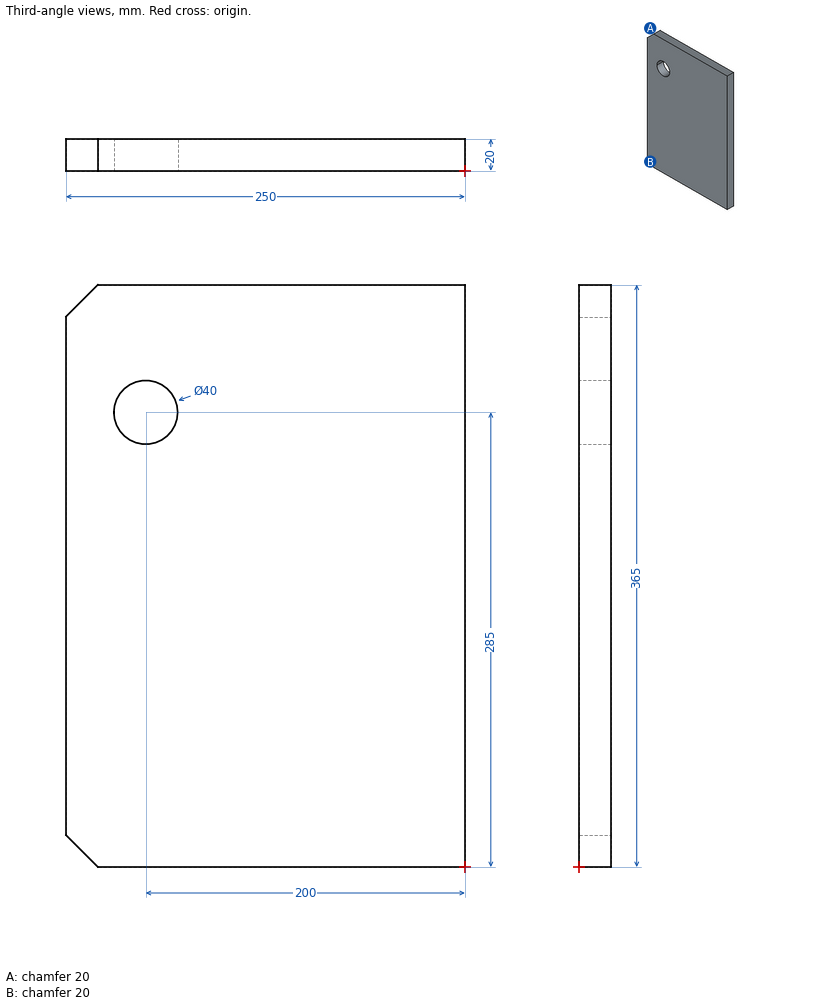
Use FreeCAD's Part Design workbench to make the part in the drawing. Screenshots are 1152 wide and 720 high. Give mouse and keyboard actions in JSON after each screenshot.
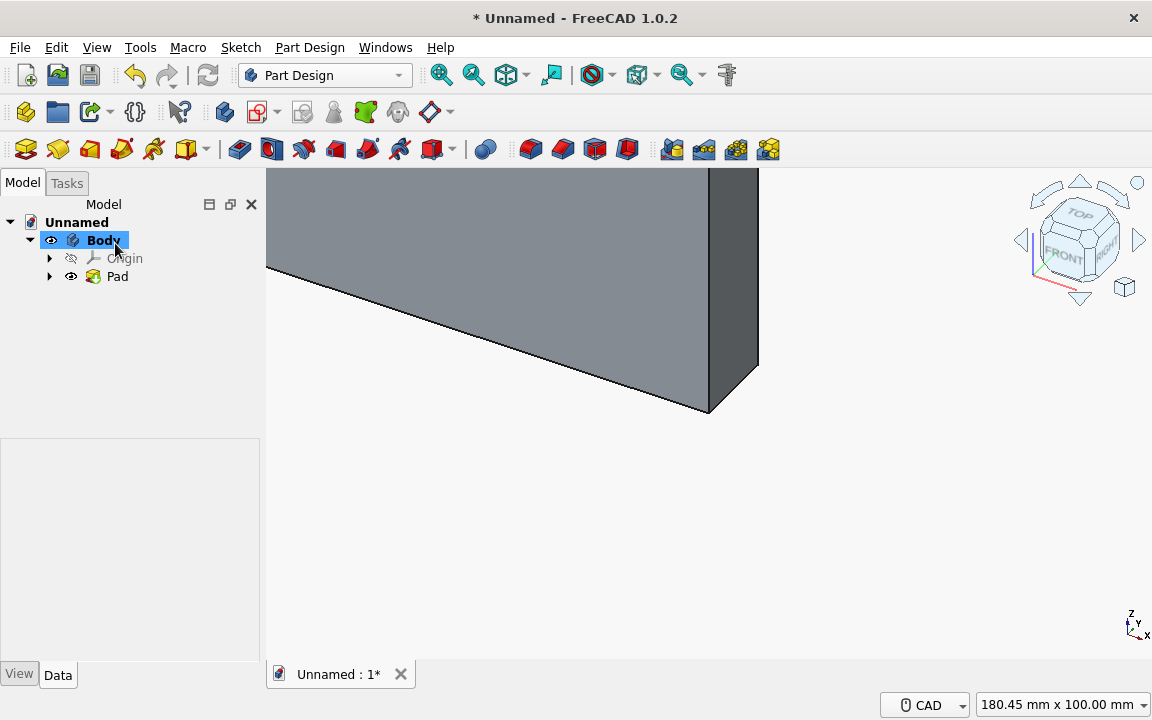
{"action": "key", "text": "v f"}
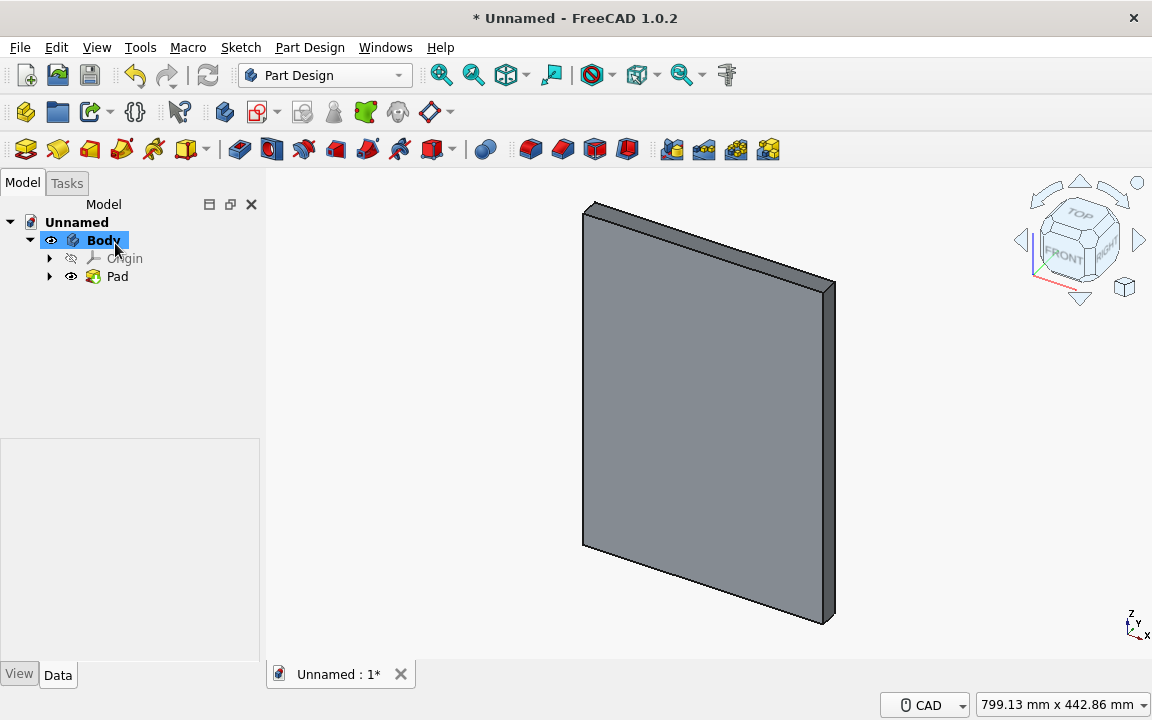
{"action": "key", "text": "0"}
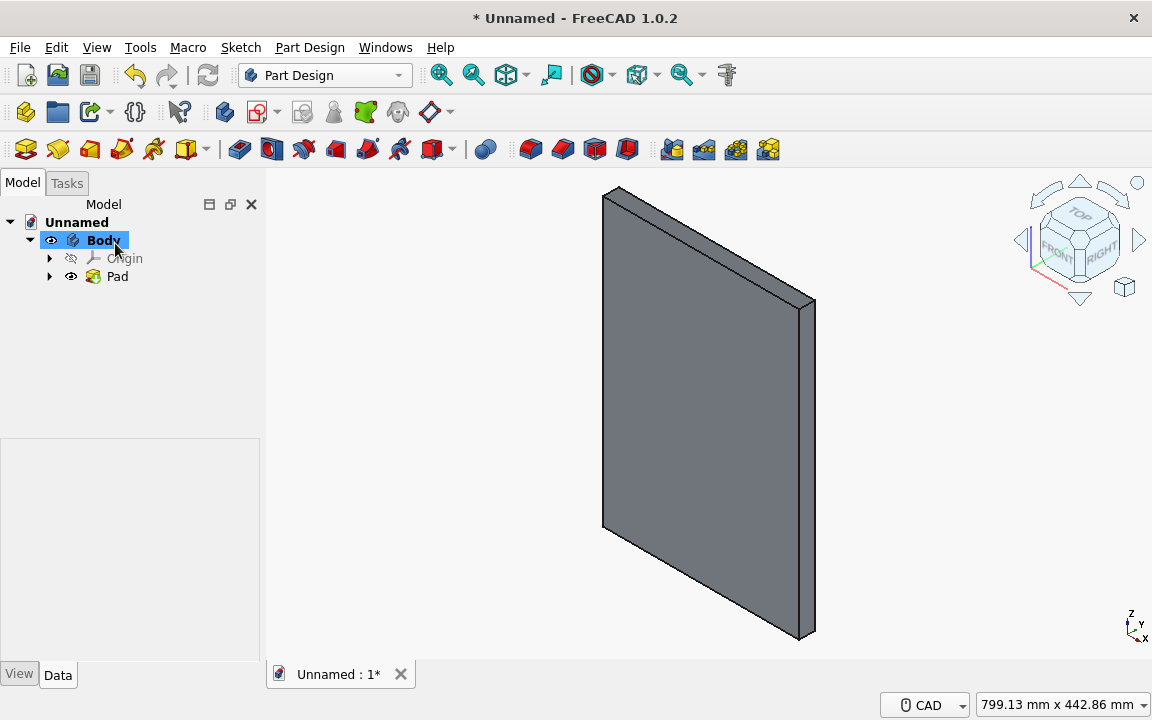
{"action": "key", "text": "2"}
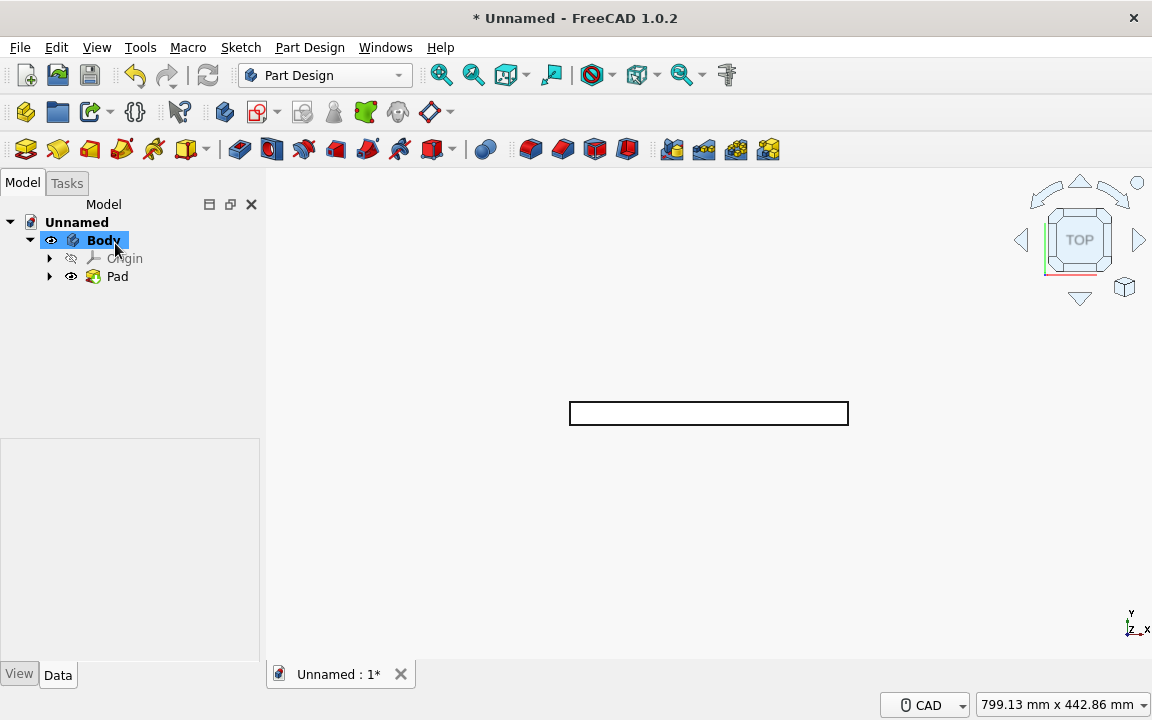
{"action": "key", "text": "v f"}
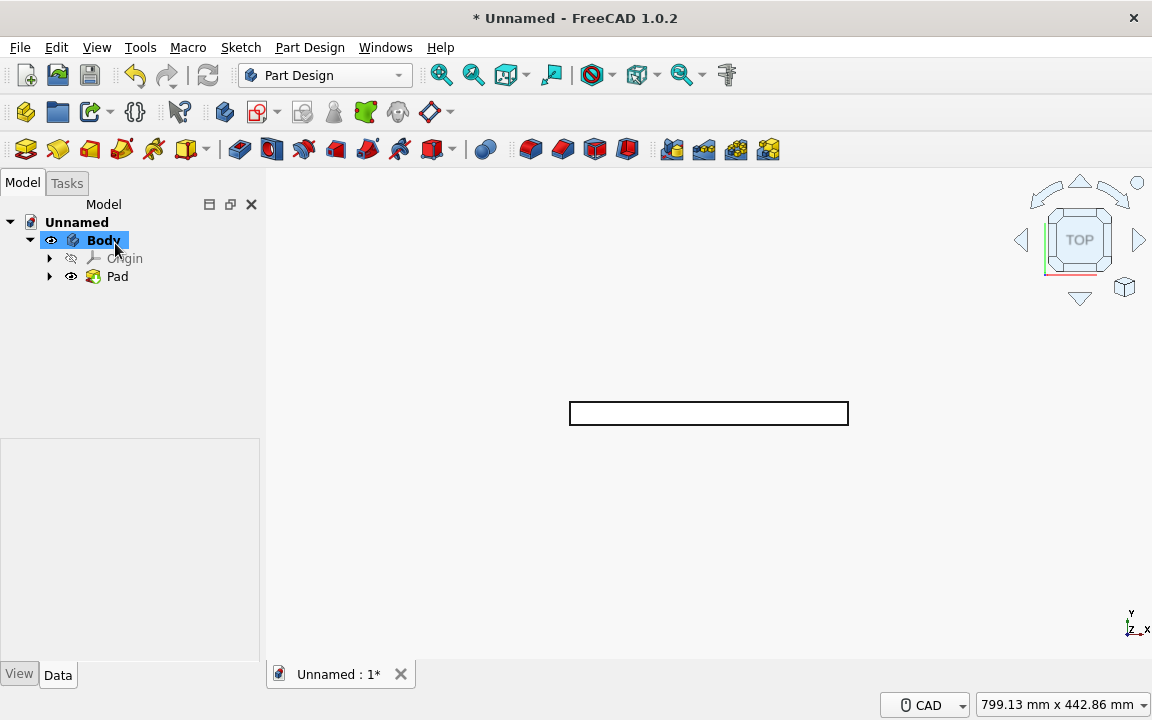
{"action": "left_click", "coordinate": [570, 412]}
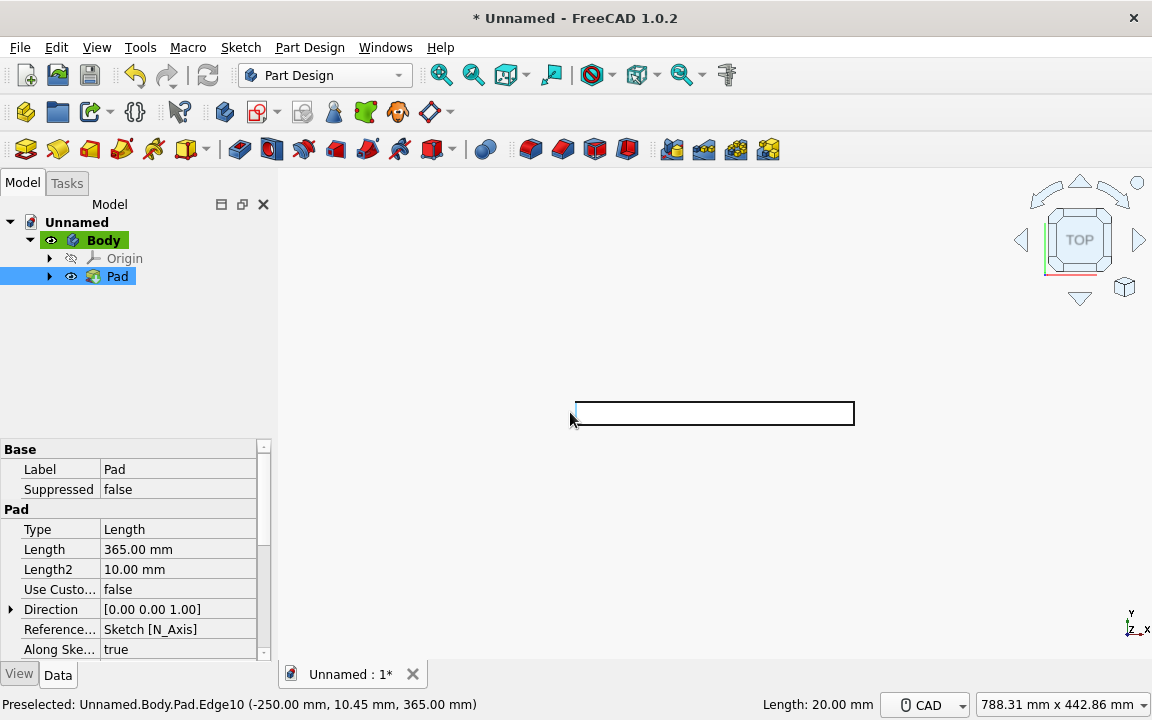
{"action": "left_click", "coordinate": [564, 150]}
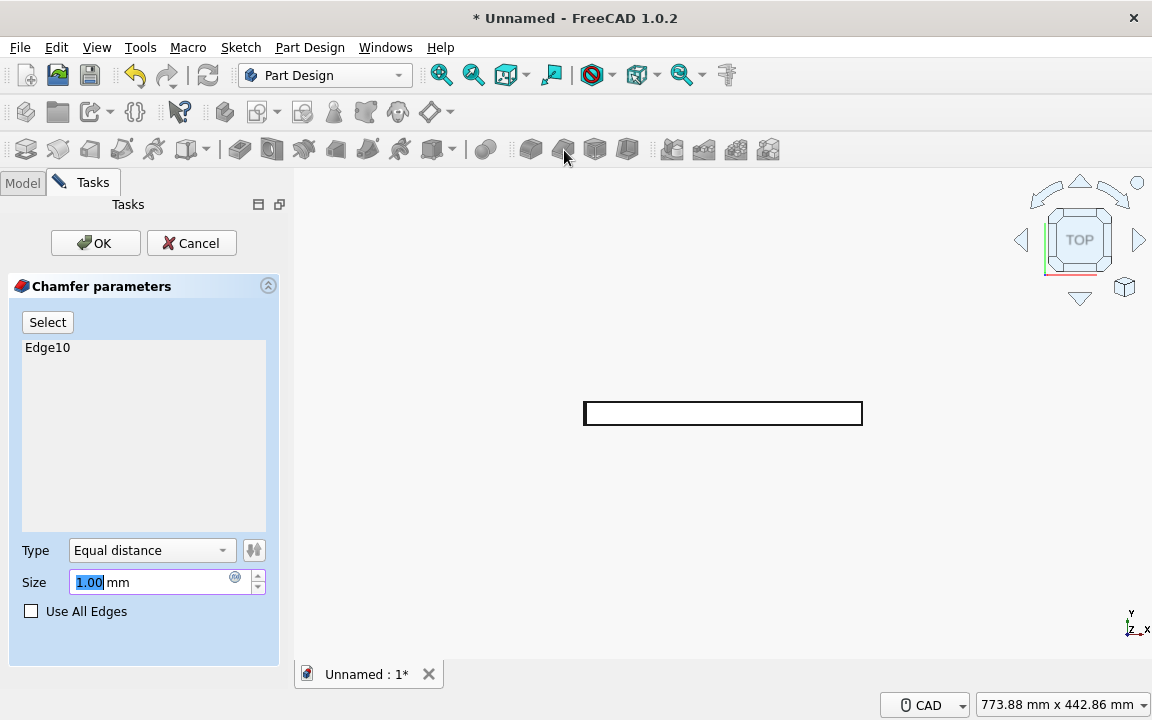
{"action": "type", "text": "20"}
{"action": "key", "text": "Tab"}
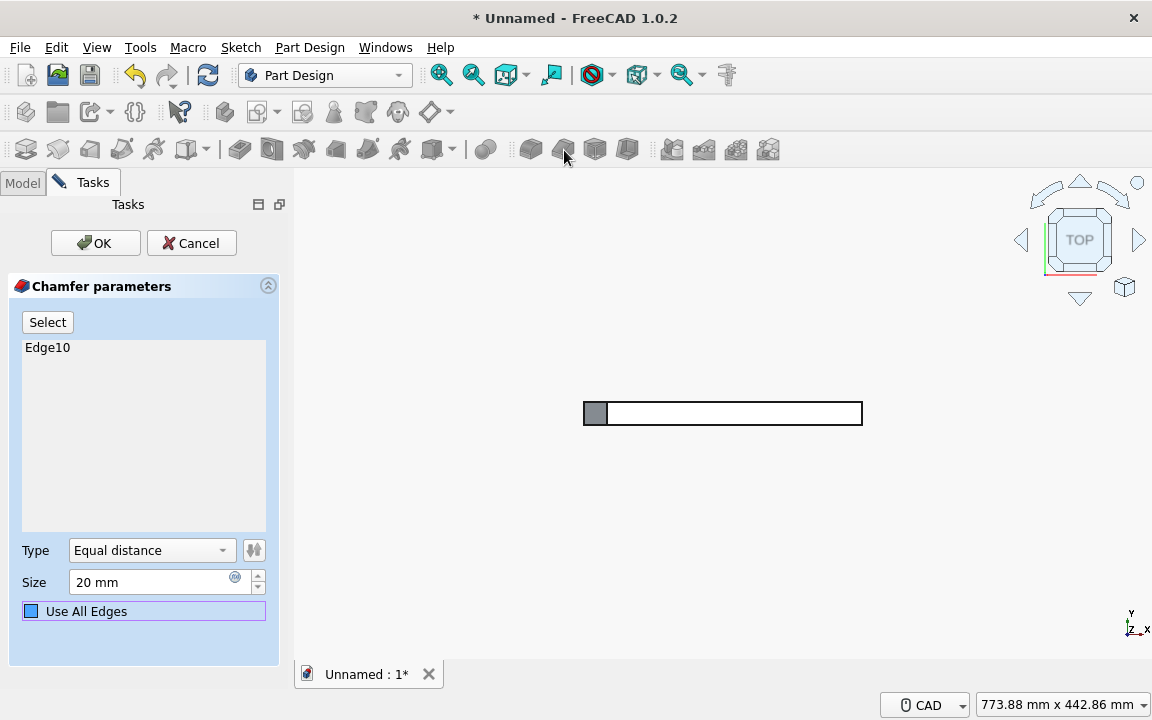
{"action": "left_click", "coordinate": [96, 243]}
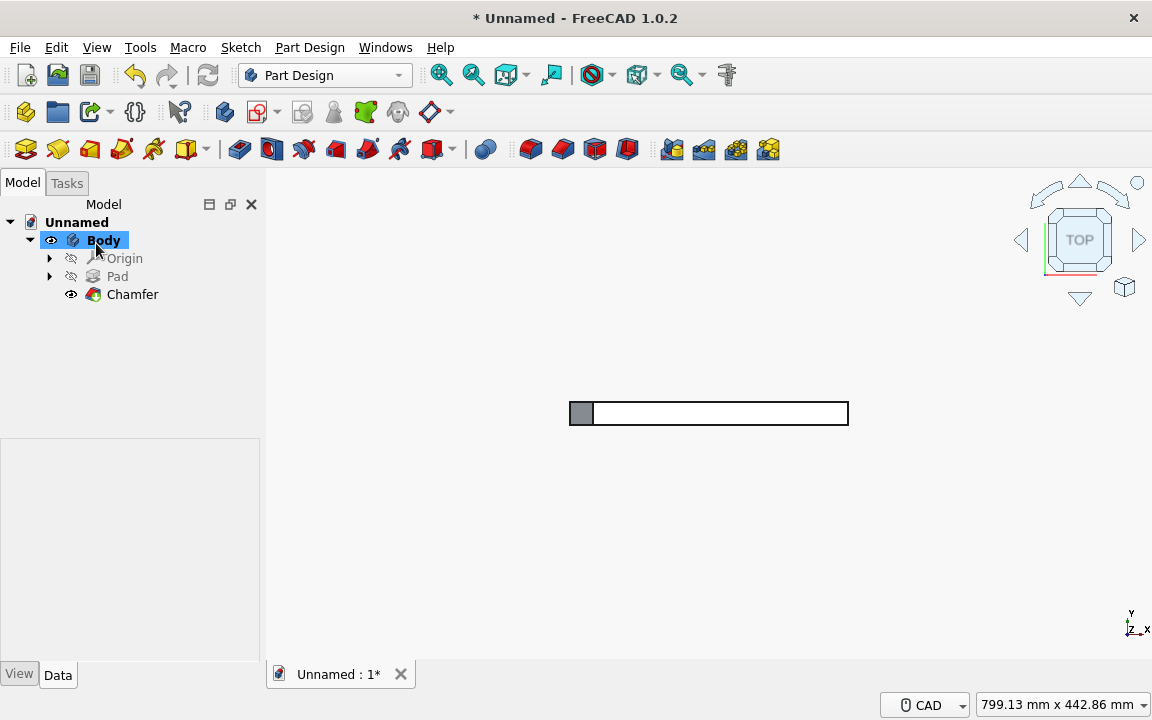
{"action": "key", "text": "v f"}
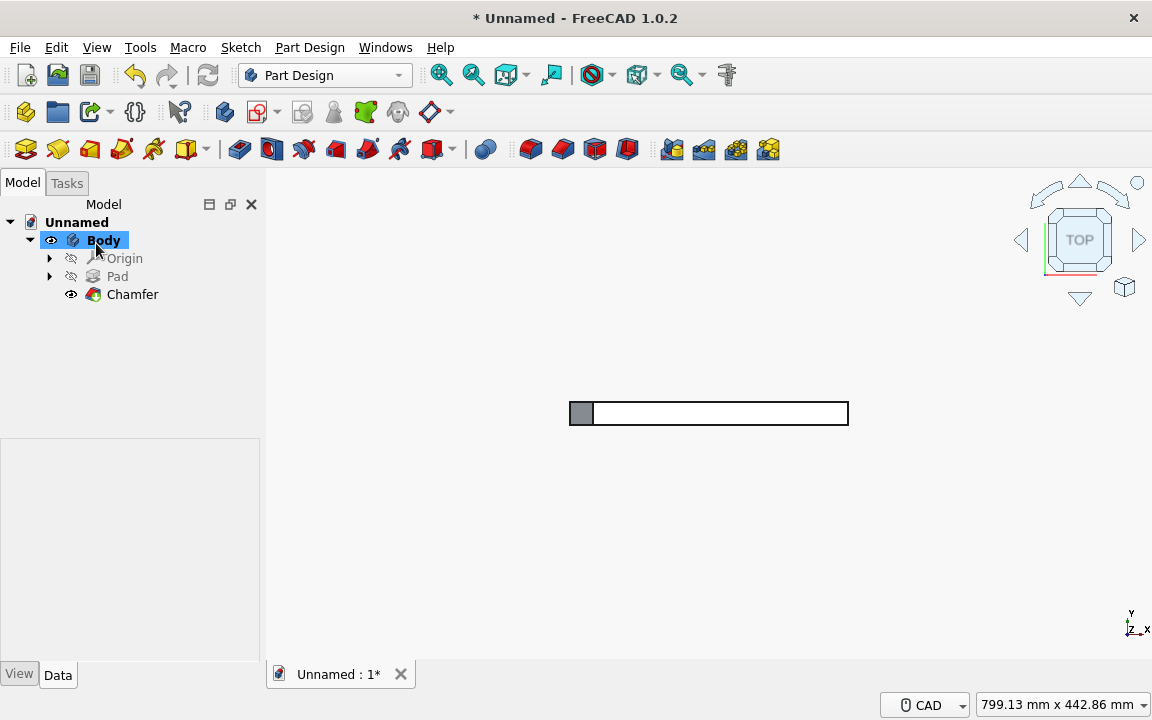
{"action": "key", "text": "4"}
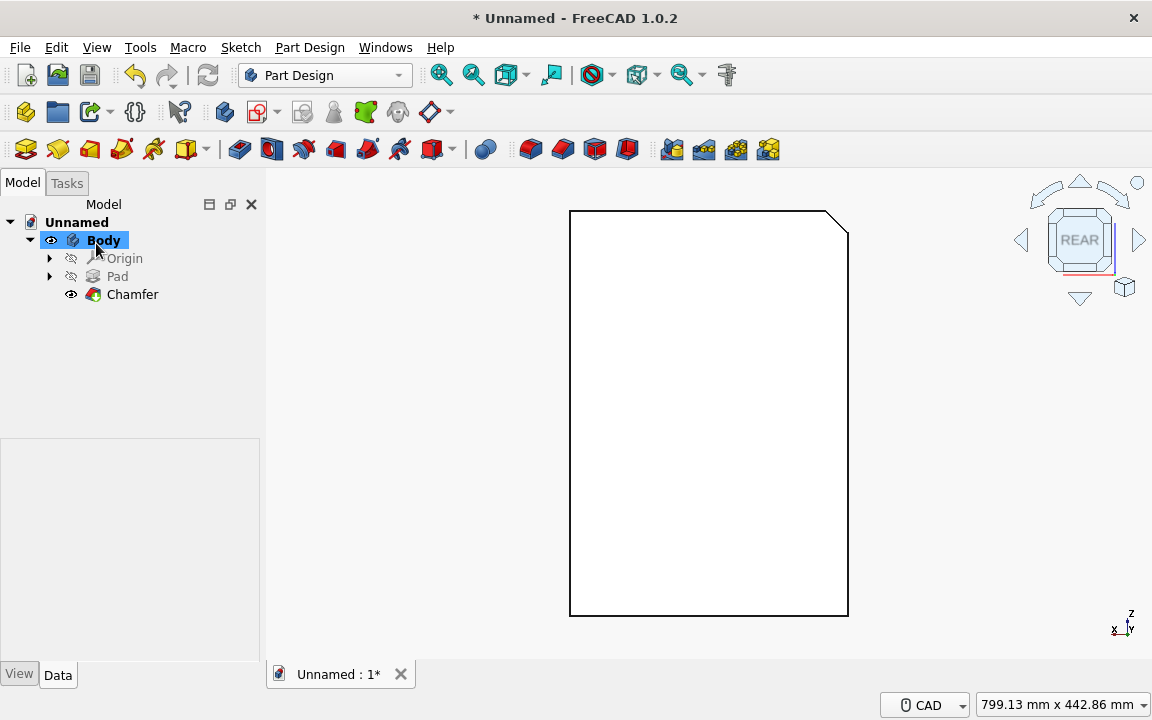
{"action": "left_click", "coordinate": [709, 355]}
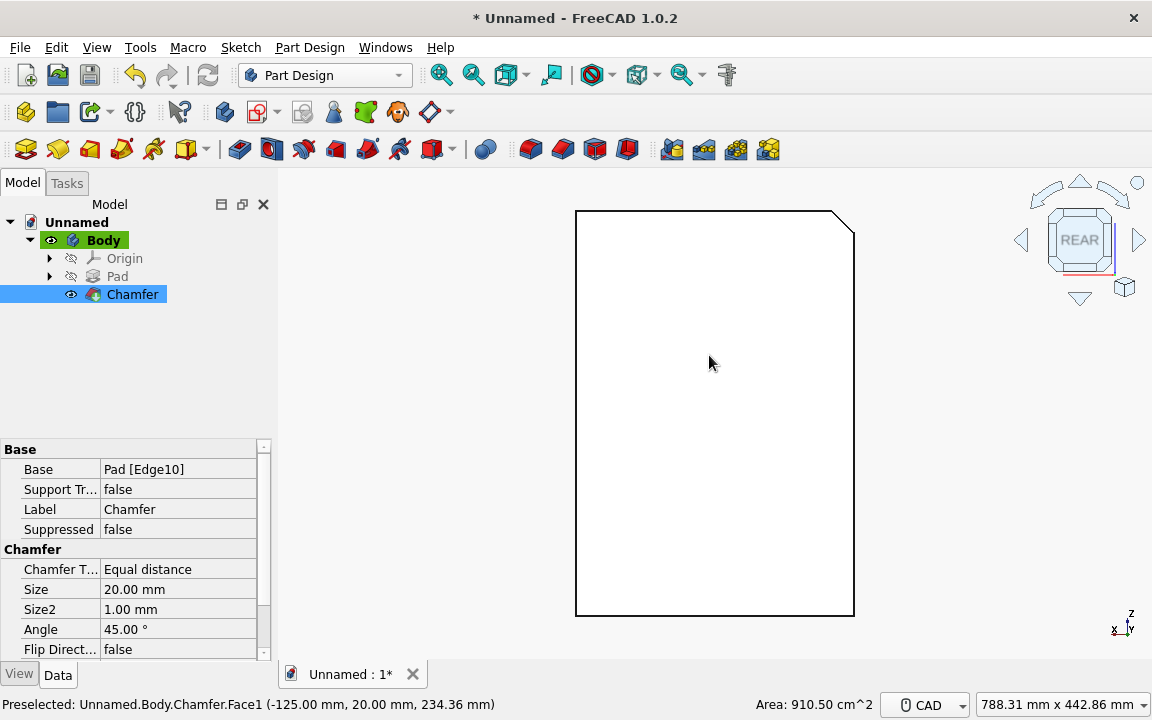
{"action": "left_click", "coordinate": [258, 112]}